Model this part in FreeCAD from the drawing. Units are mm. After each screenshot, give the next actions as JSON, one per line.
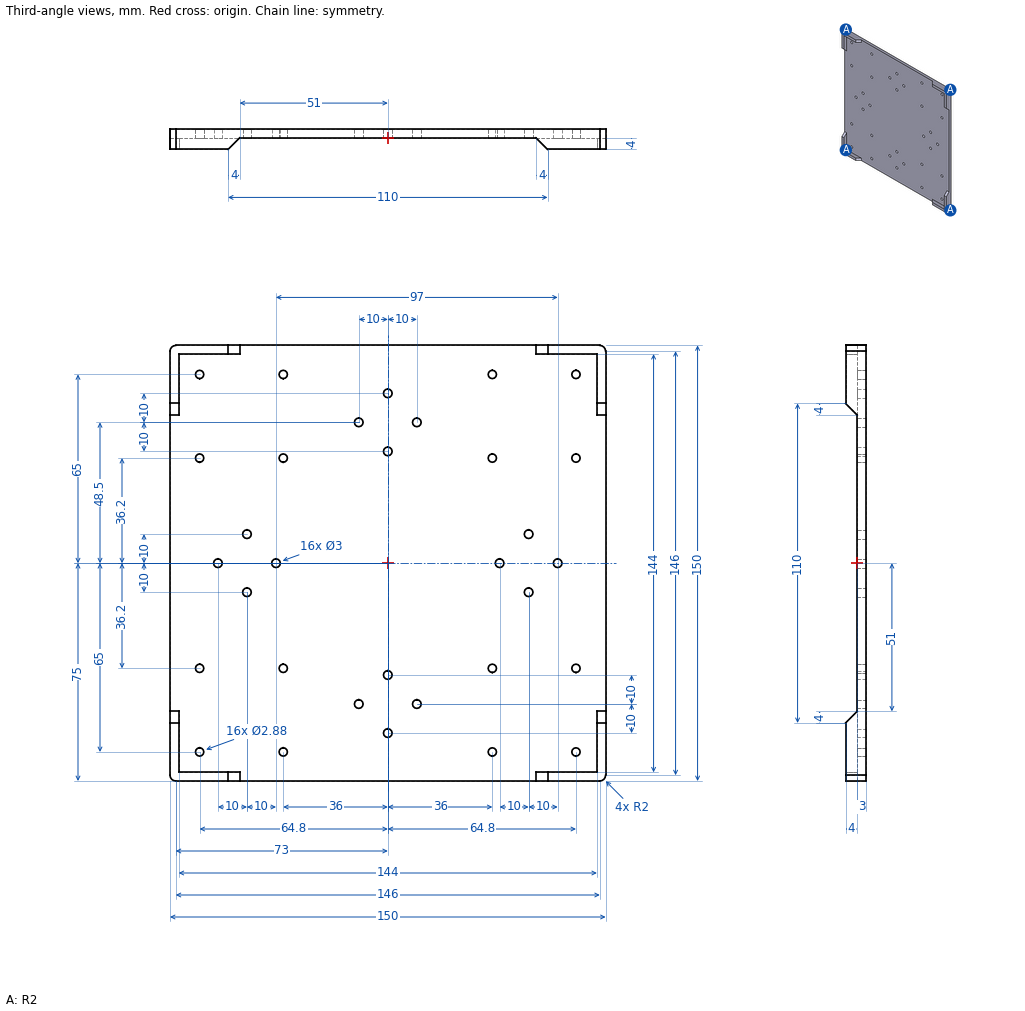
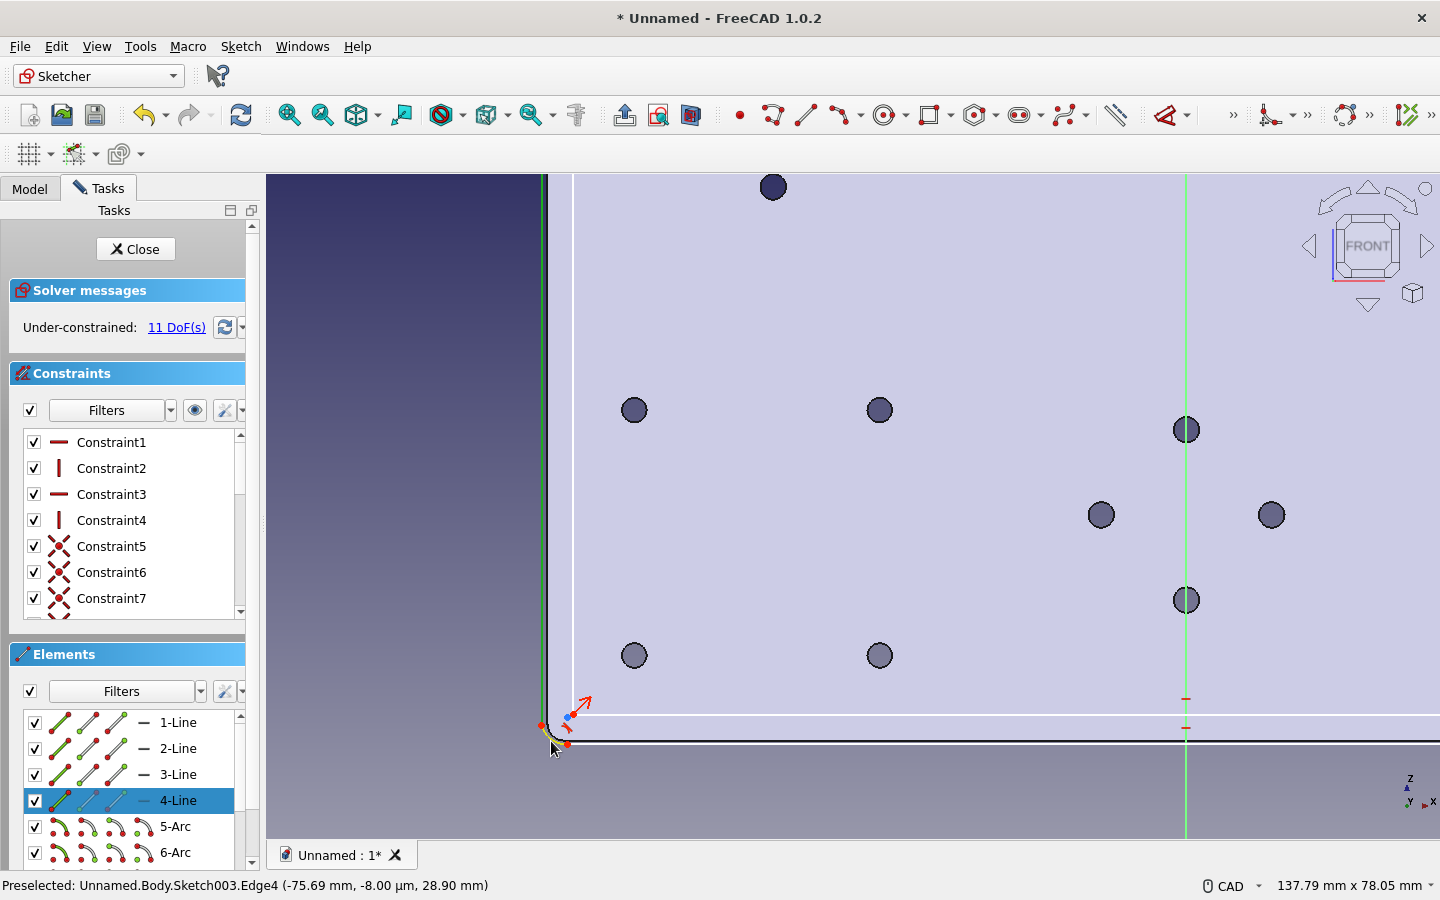
{"action": "left_click", "coordinate": [551, 739]}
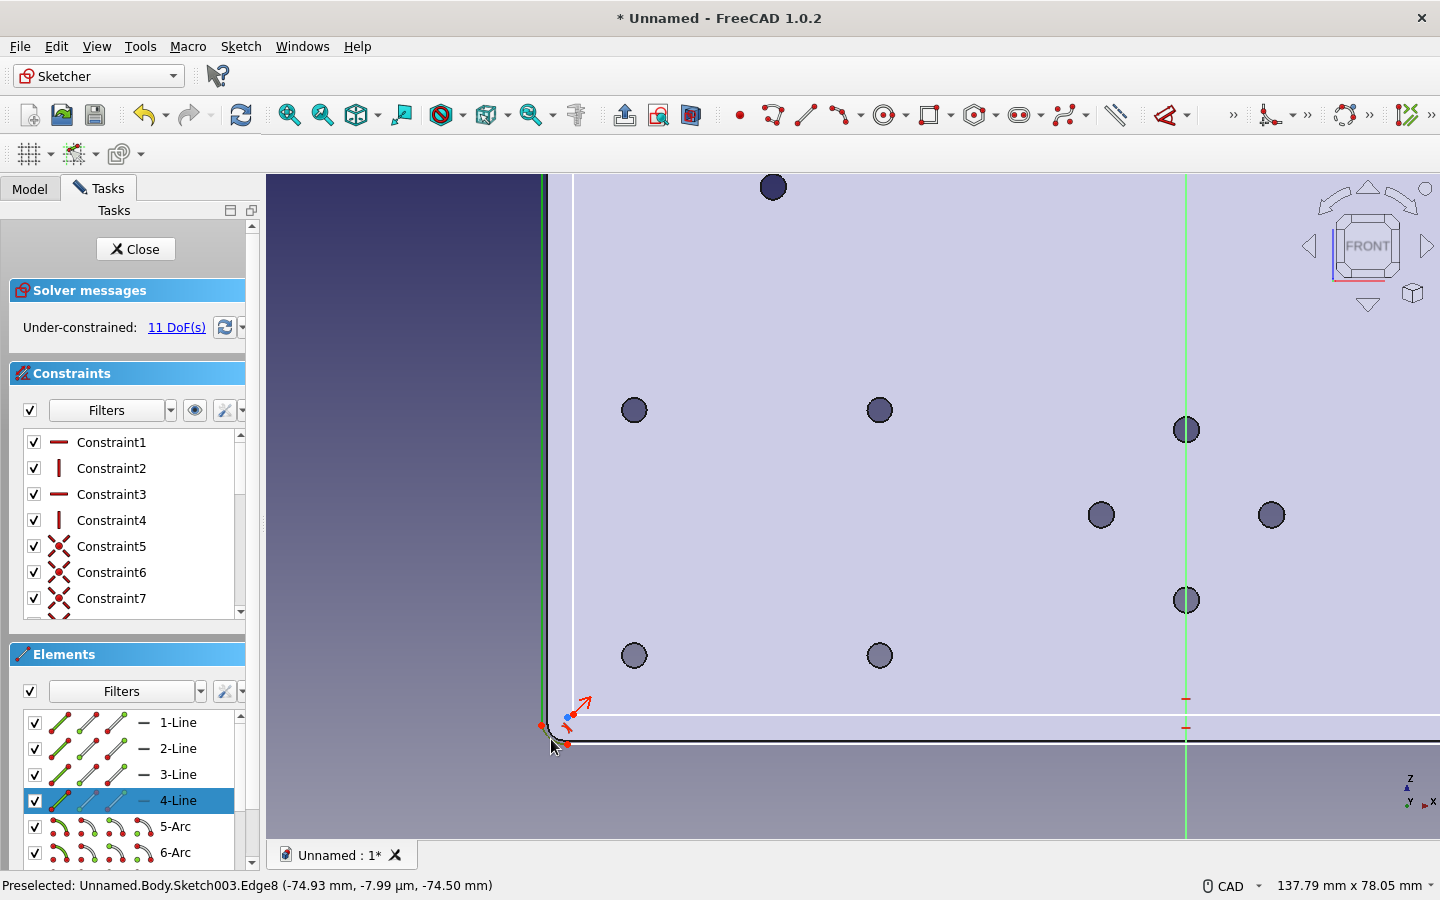
{"action": "key", "text": "t"}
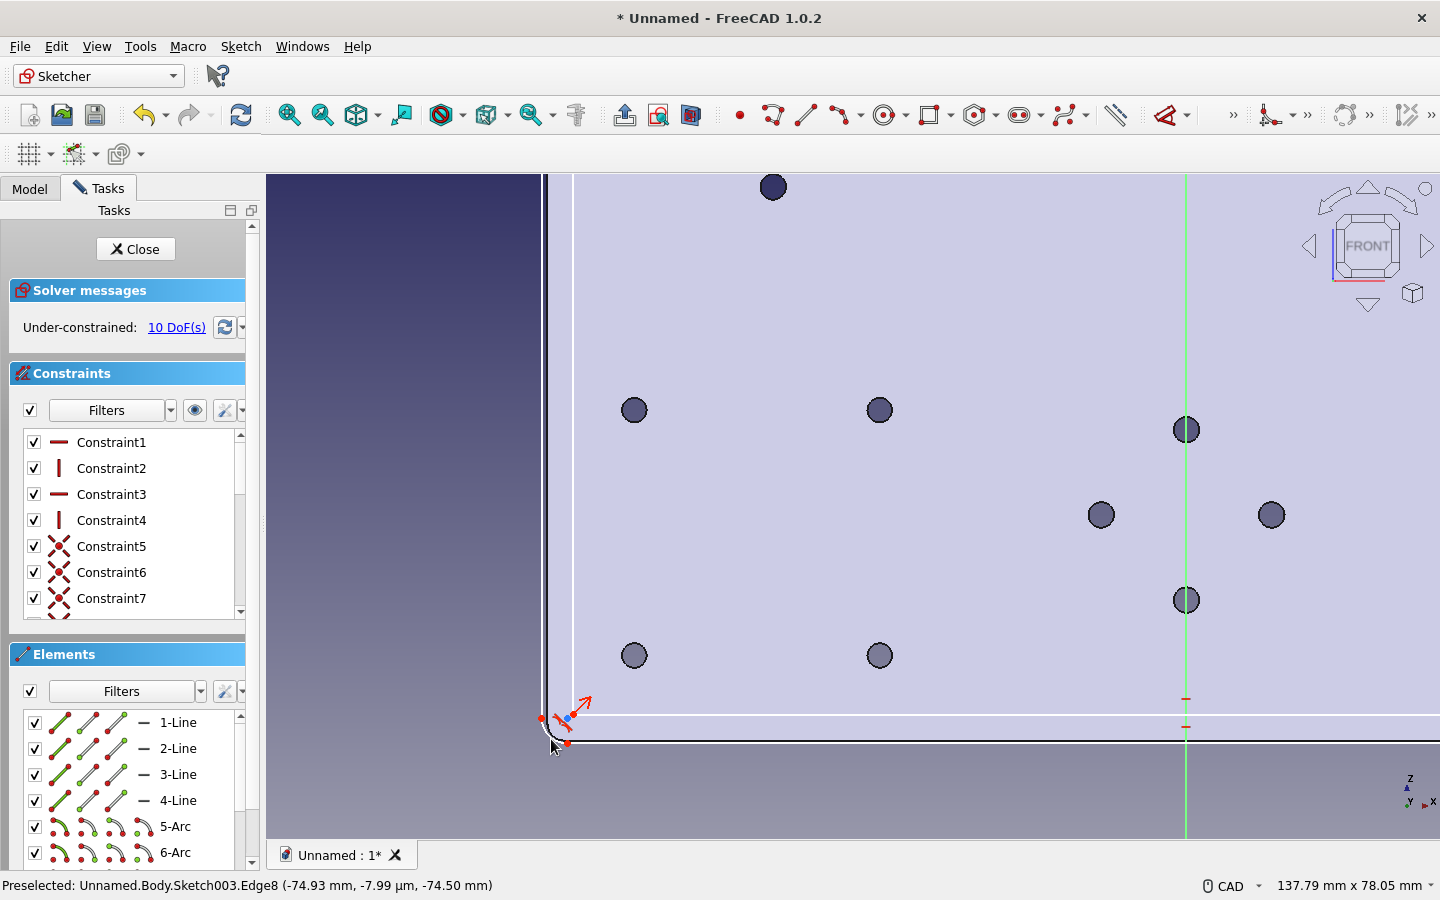
{"action": "scroll", "coordinate": [551, 742], "scroll_direction": "down", "scroll_amount": 5}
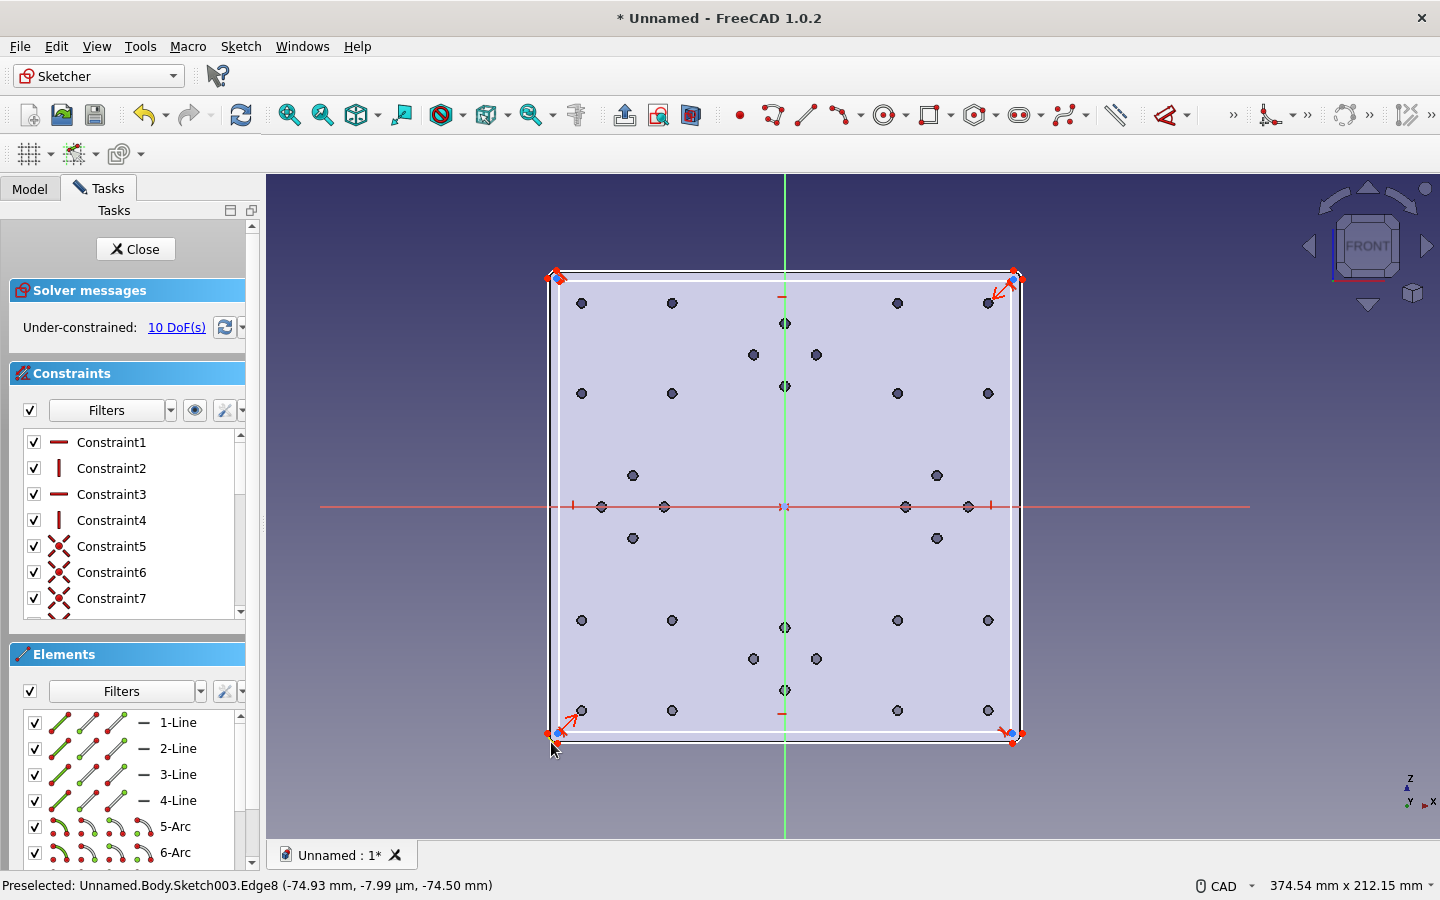
{"action": "scroll", "coordinate": [1017, 742], "scroll_direction": "up", "scroll_amount": 6}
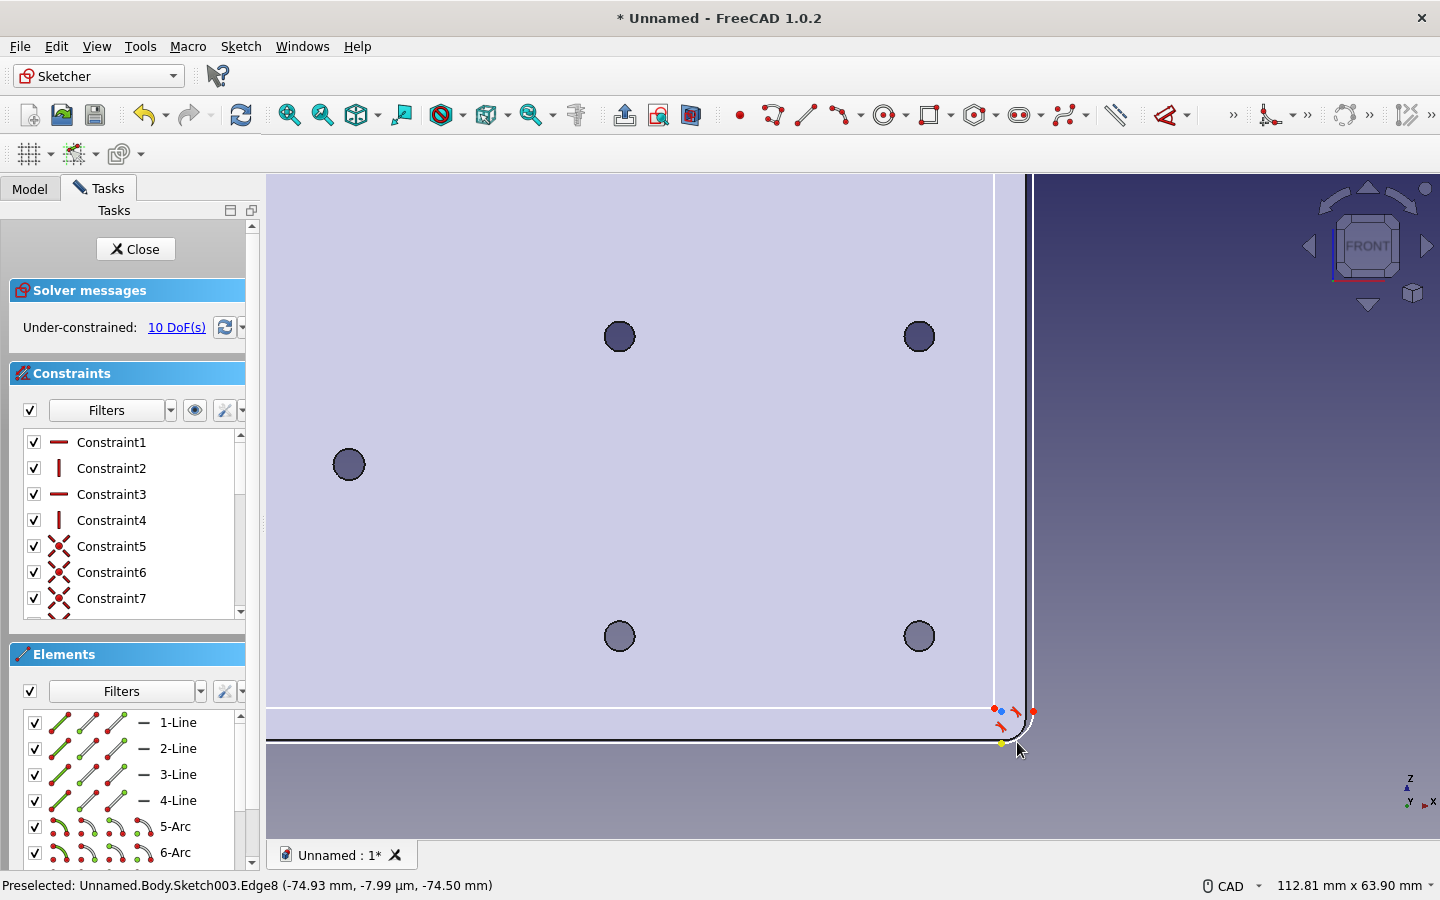
{"action": "left_click", "coordinate": [1016, 740]}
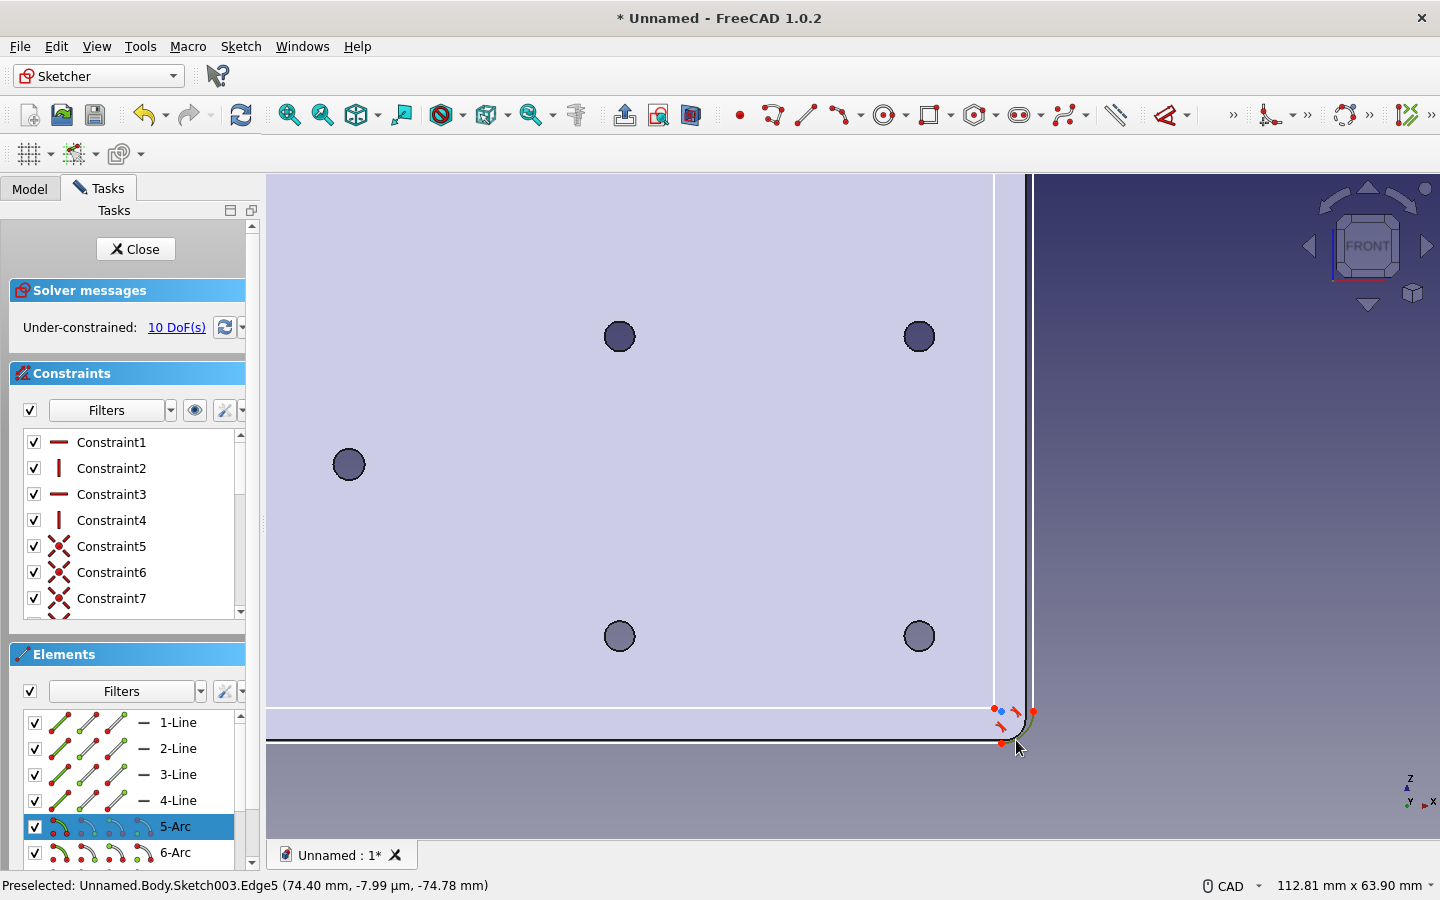
{"action": "scroll", "coordinate": [1017, 742], "scroll_direction": "down", "scroll_amount": 6}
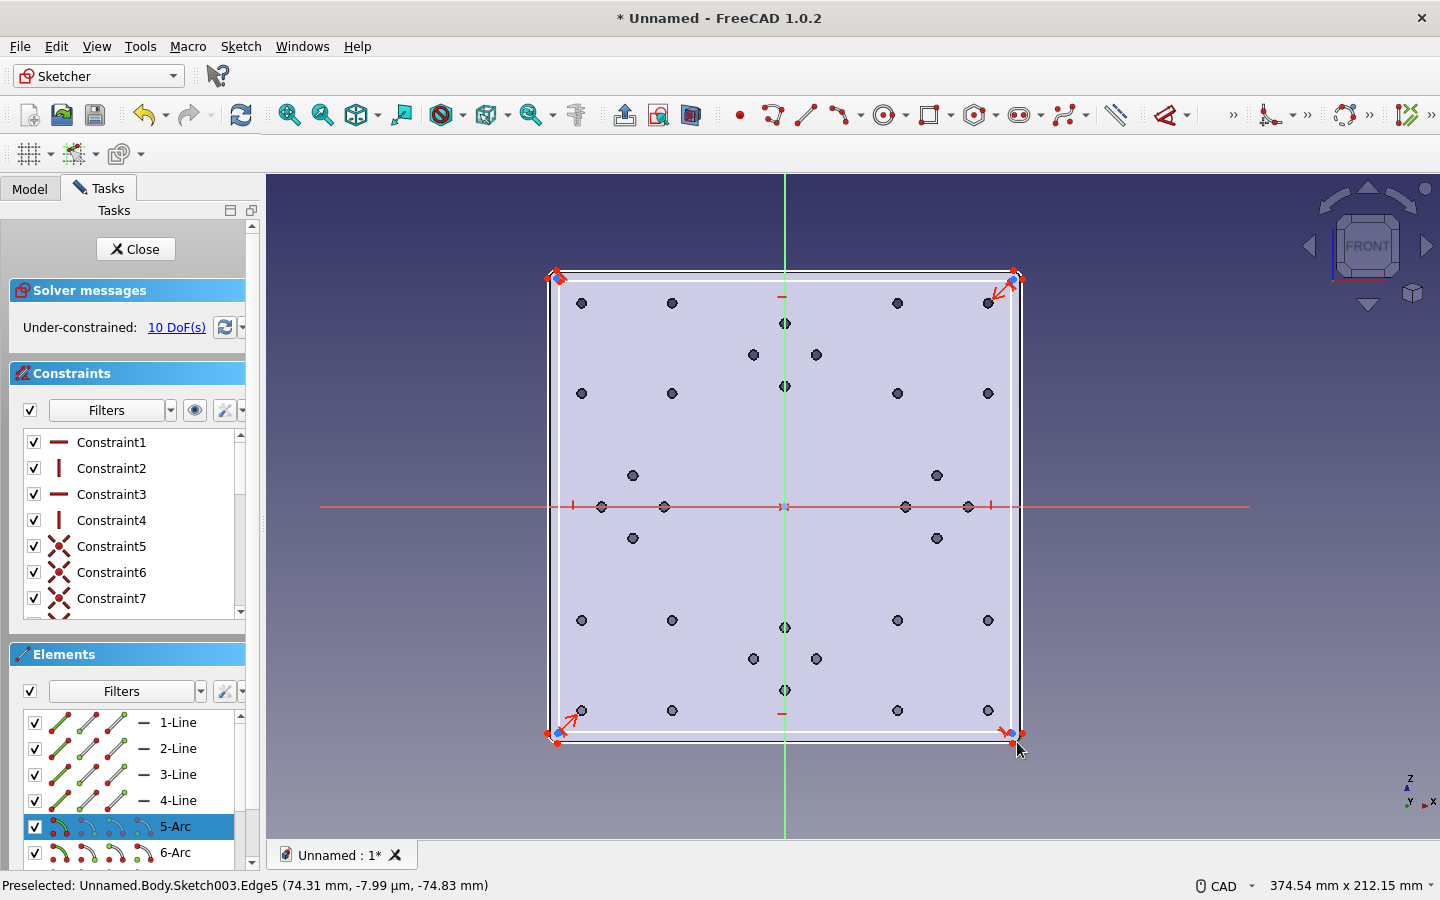
{"action": "scroll", "coordinate": [1021, 275], "scroll_direction": "up", "scroll_amount": 7}